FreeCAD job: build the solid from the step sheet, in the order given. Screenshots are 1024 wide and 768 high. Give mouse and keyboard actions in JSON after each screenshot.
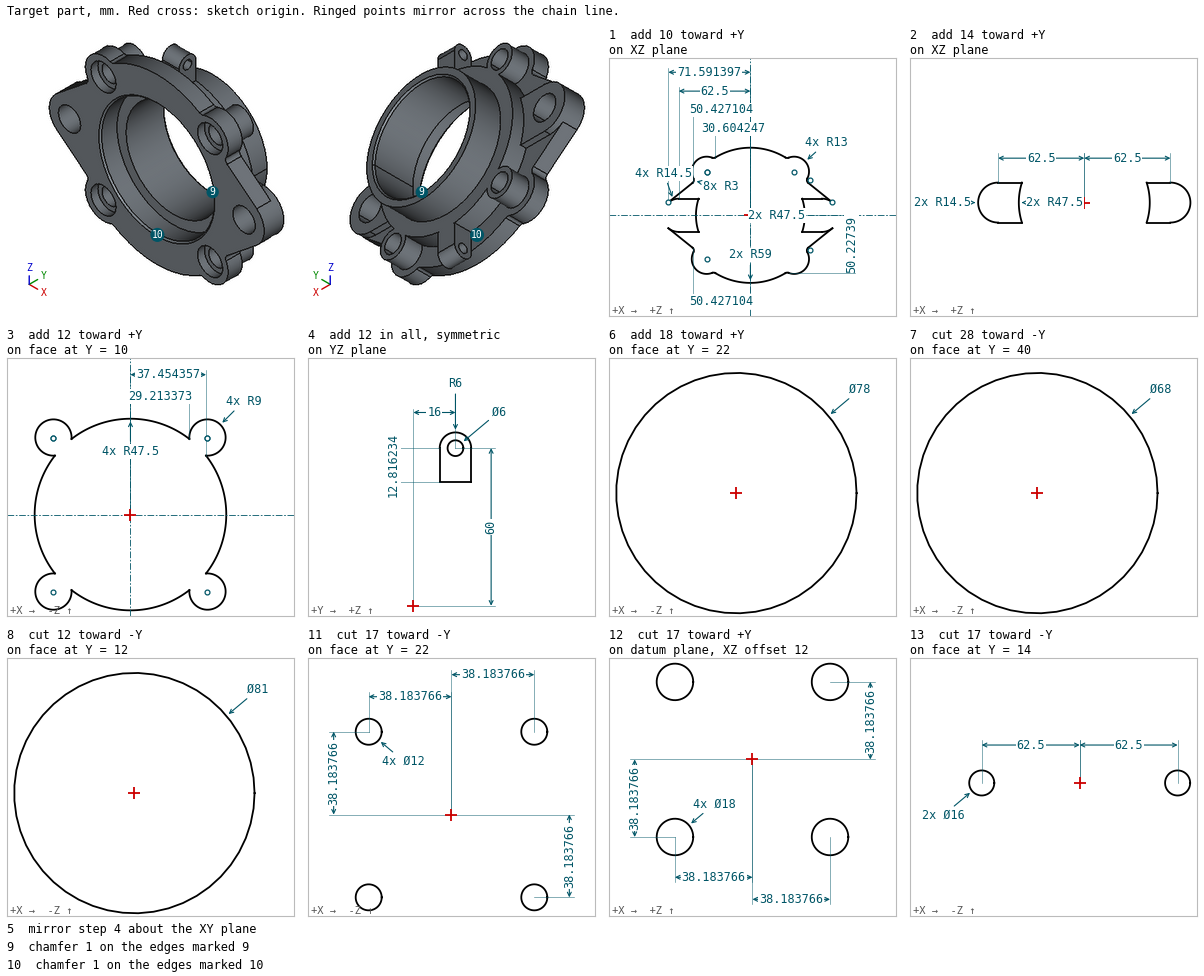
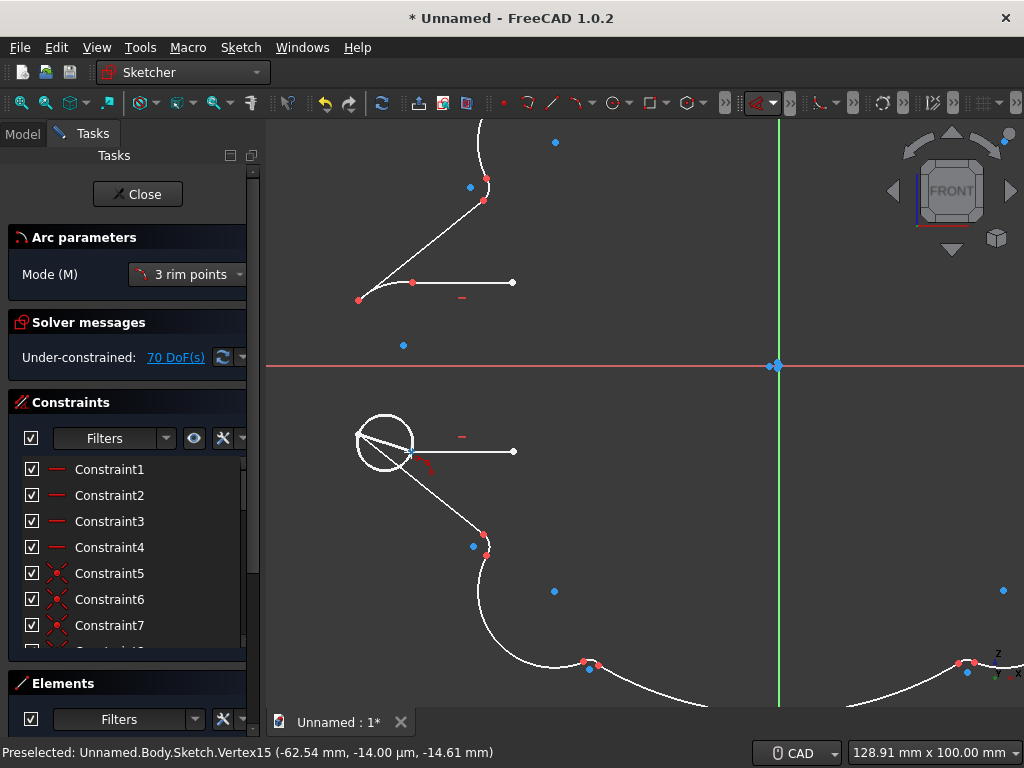
{"action": "scroll", "coordinate": [383, 446], "scroll_direction": "up", "scroll_amount": 6}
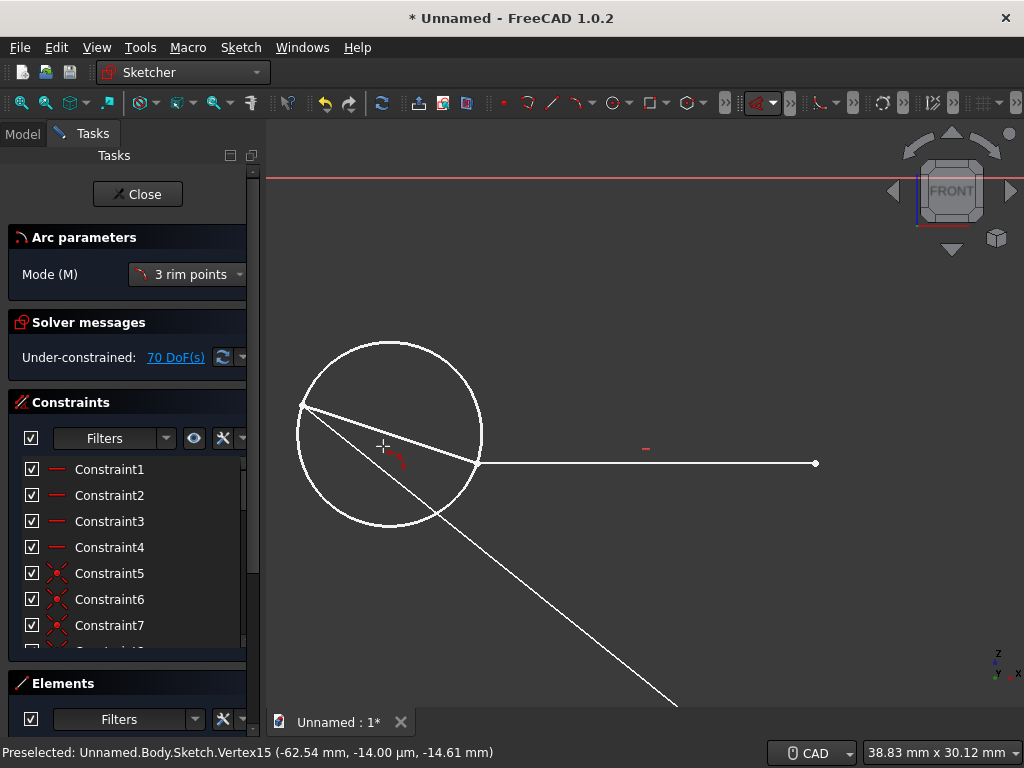
{"action": "left_click", "coordinate": [384, 445]}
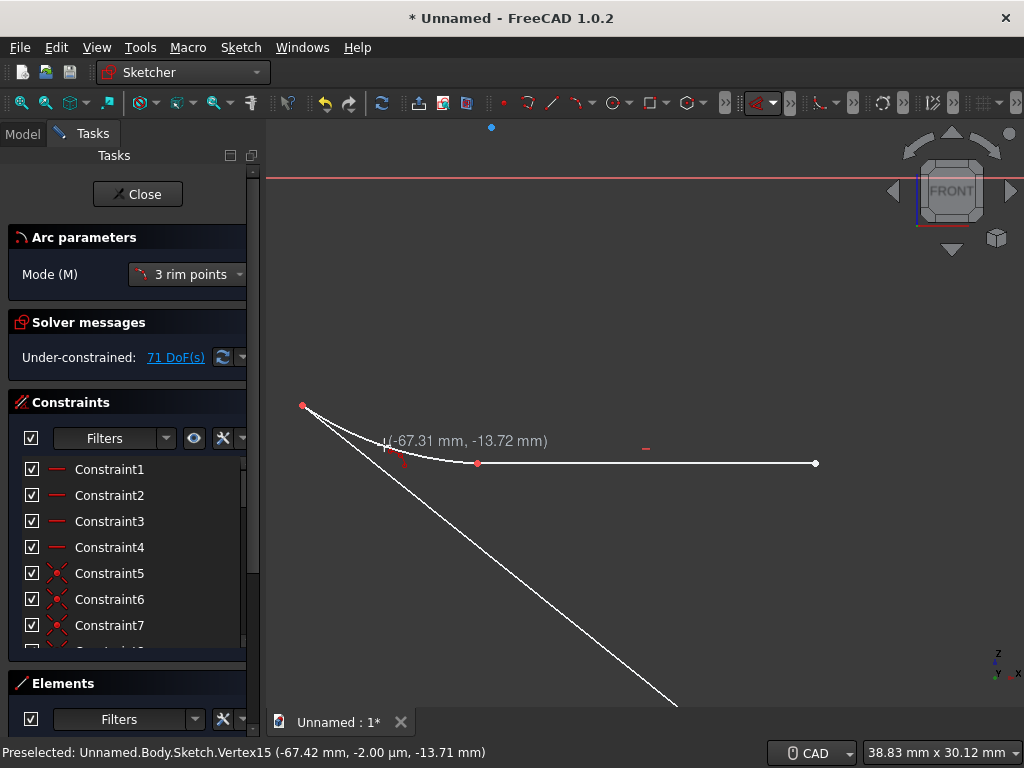
{"action": "scroll", "coordinate": [401, 450], "scroll_direction": "down", "scroll_amount": 10}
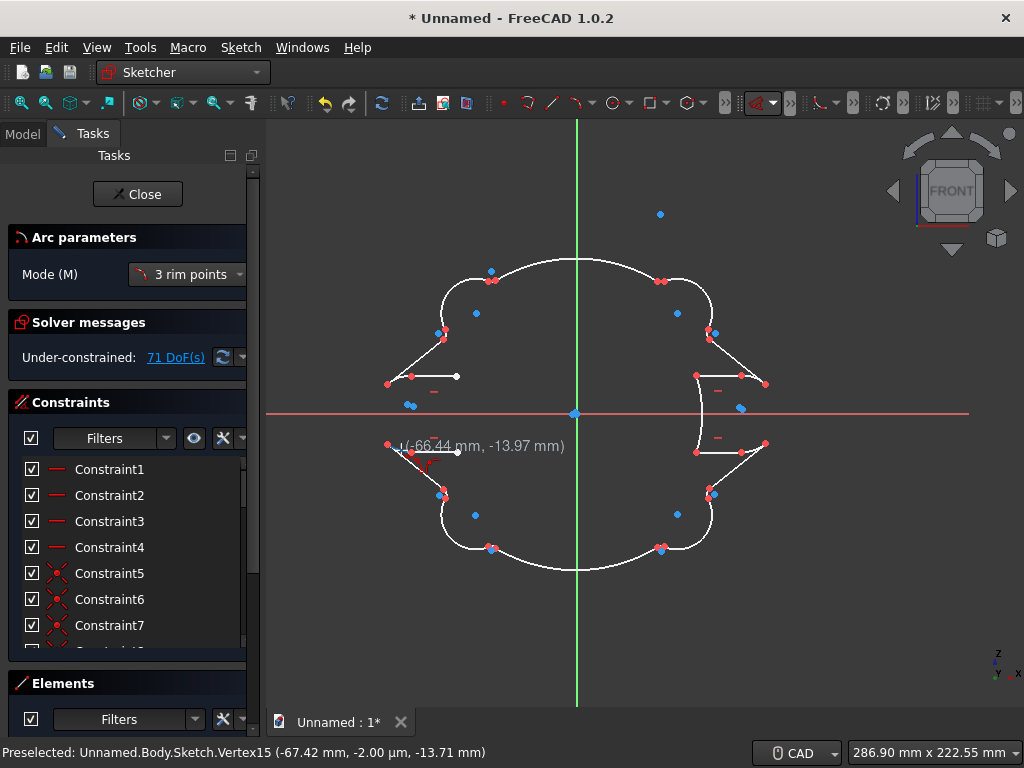
{"action": "left_click", "coordinate": [457, 452]}
{"action": "left_click", "coordinate": [457, 376]}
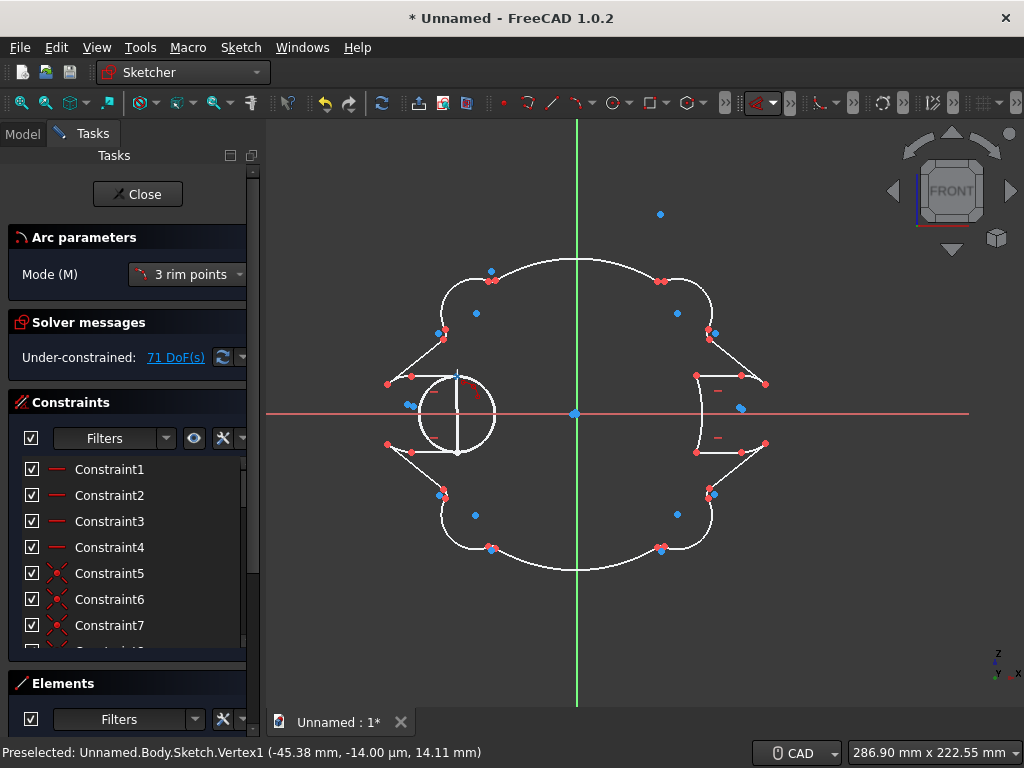
{"action": "scroll", "coordinate": [451, 421], "scroll_direction": "up", "scroll_amount": 6}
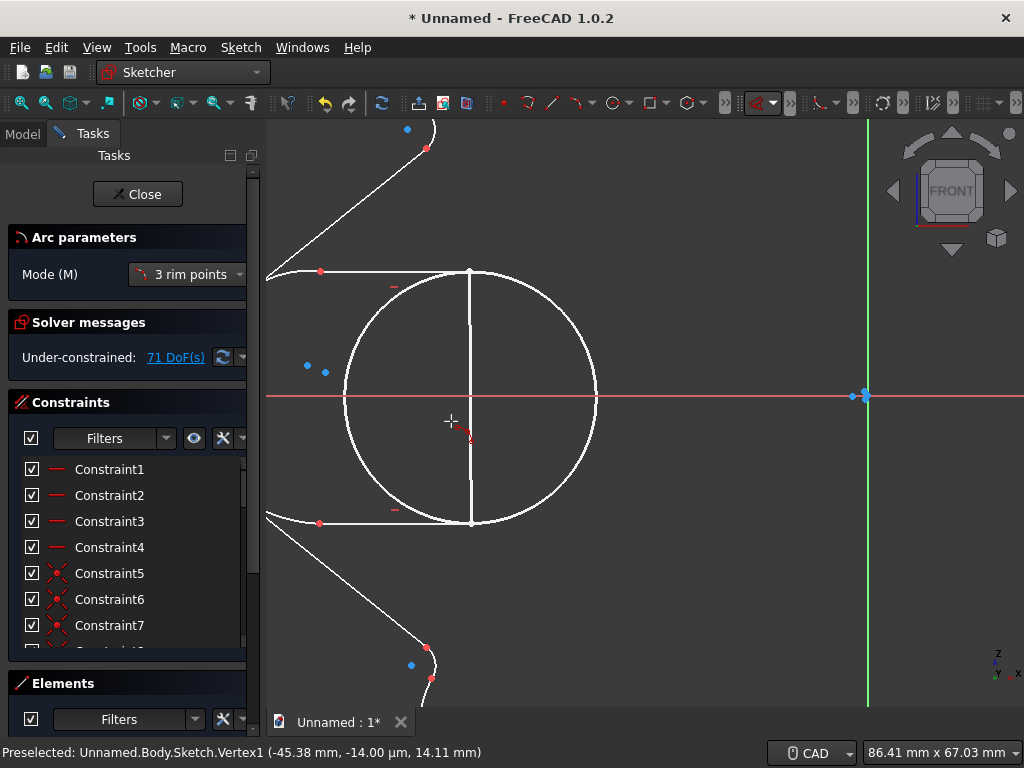
{"action": "left_click", "coordinate": [452, 421]}
{"action": "key", "text": "Escape"}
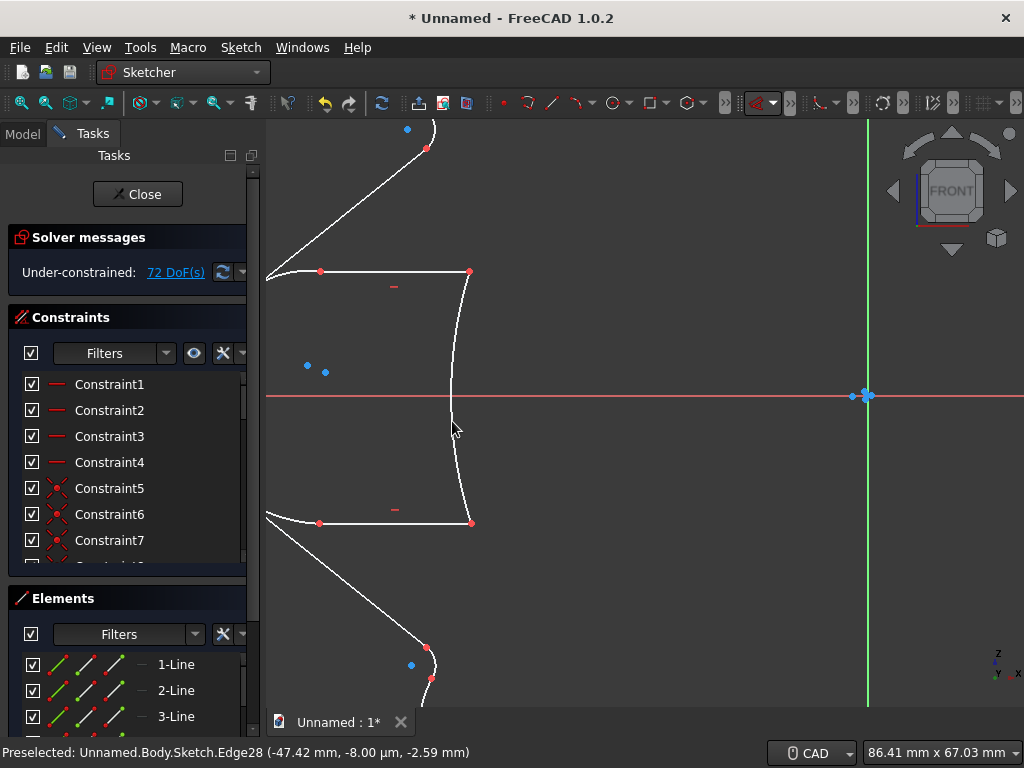
{"action": "left_click", "coordinate": [425, 272]}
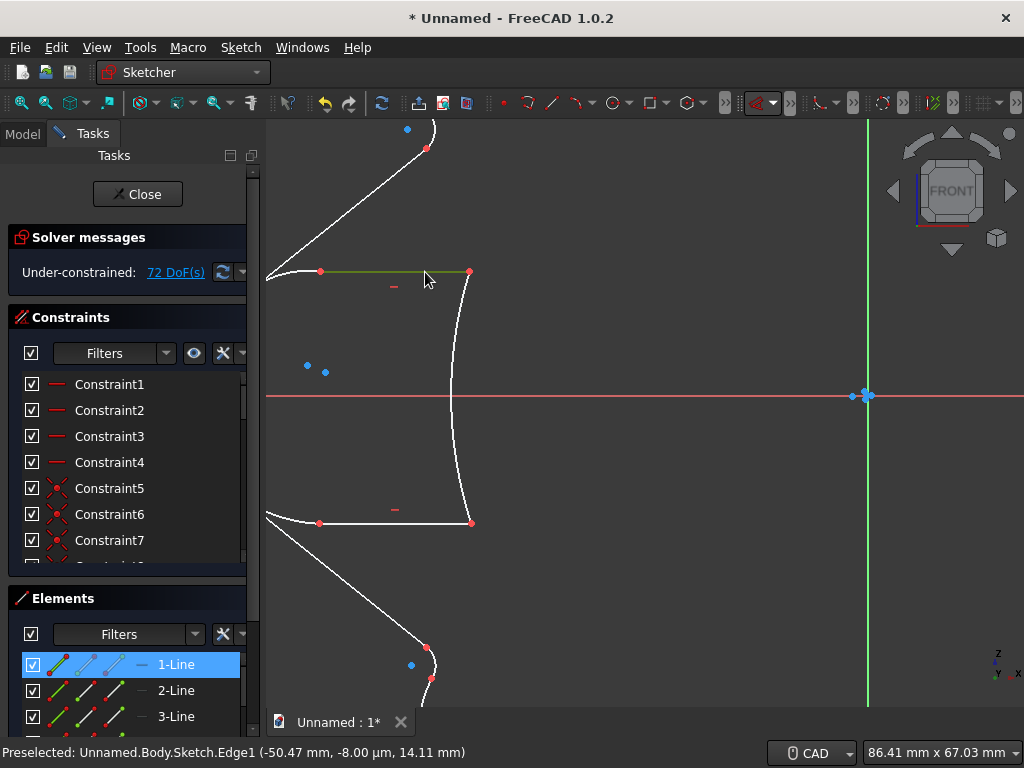
{"action": "left_click", "coordinate": [294, 272]}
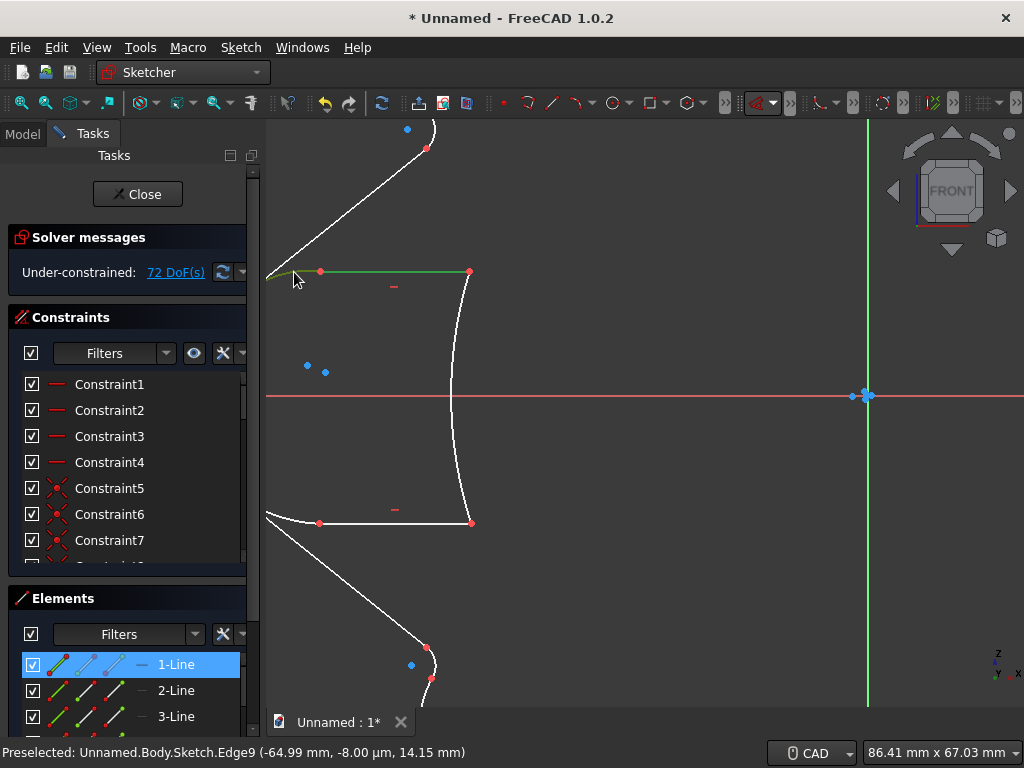
{"action": "key", "text": "t"}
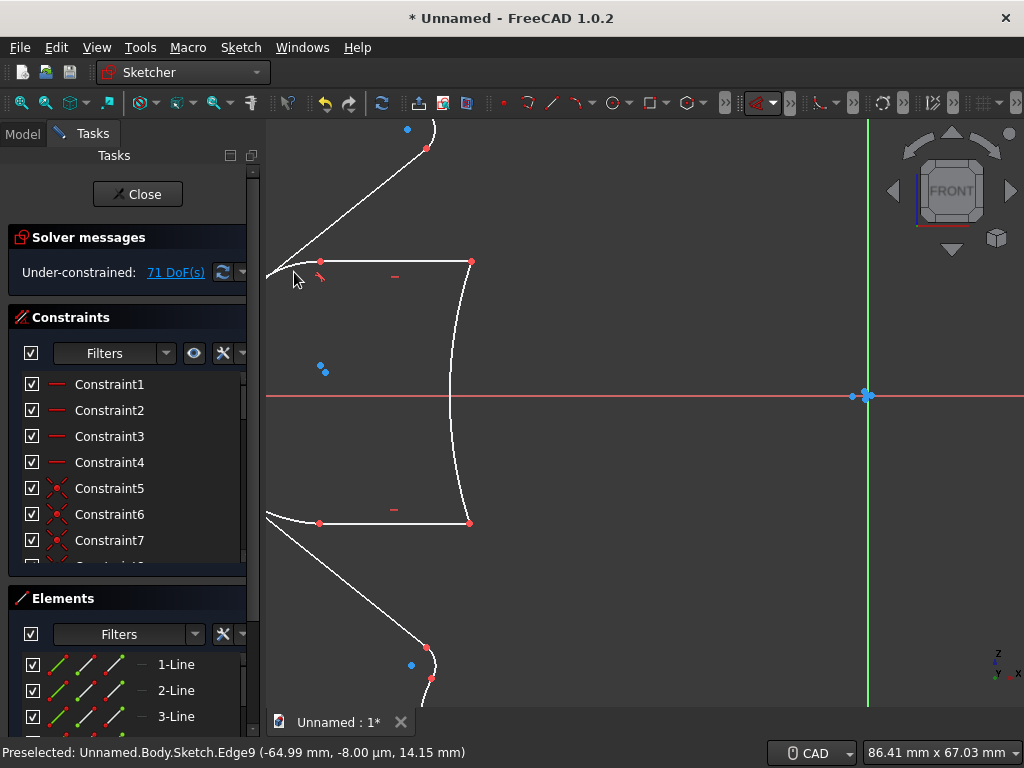
{"action": "scroll", "coordinate": [296, 254], "scroll_direction": "up", "scroll_amount": 2}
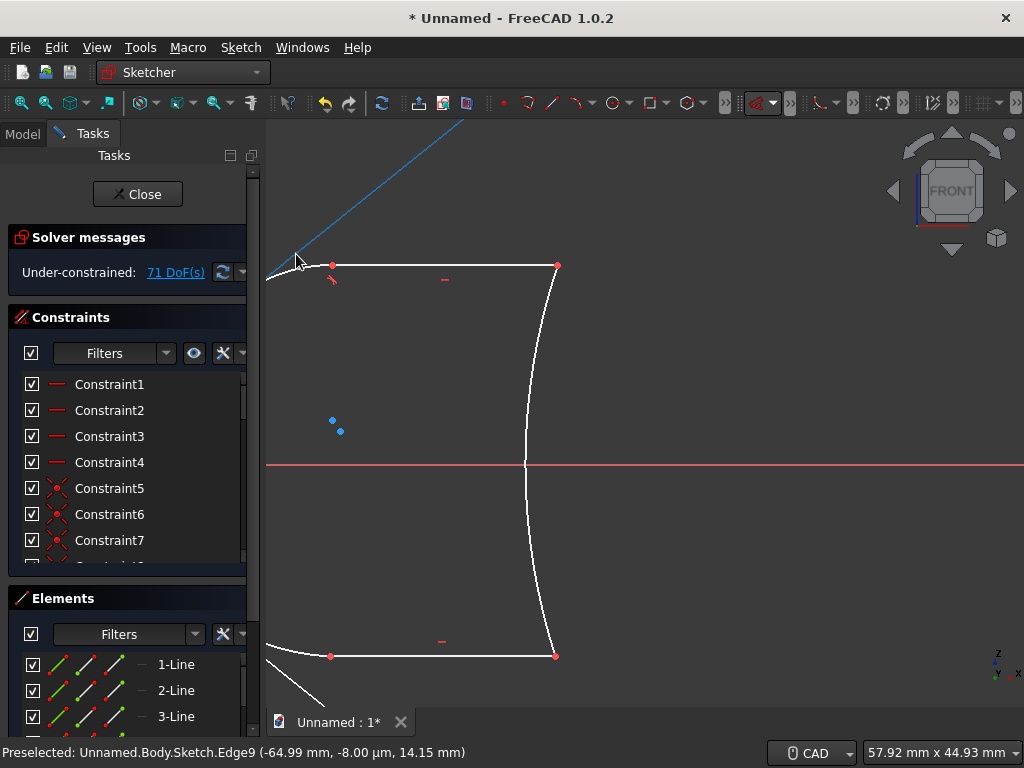
{"action": "left_click", "coordinate": [297, 253]}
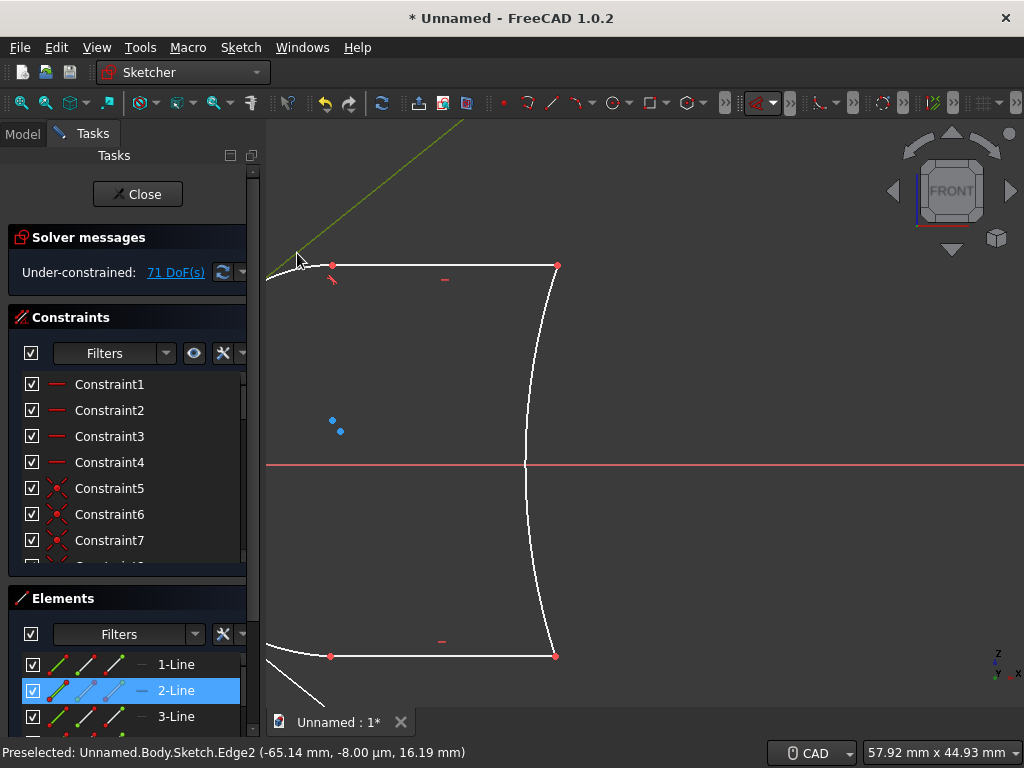
{"action": "left_click", "coordinate": [305, 267]}